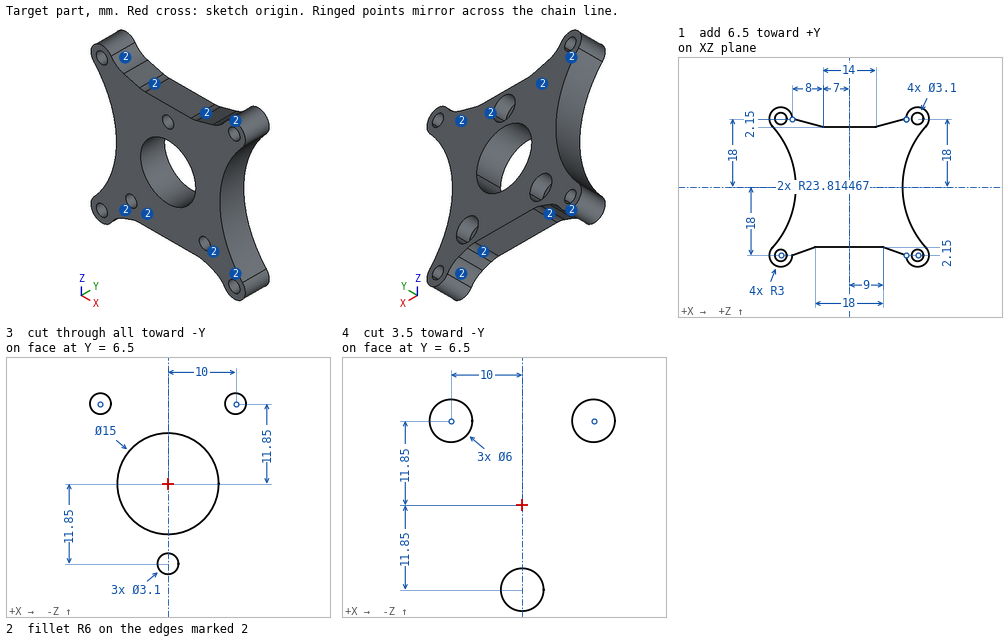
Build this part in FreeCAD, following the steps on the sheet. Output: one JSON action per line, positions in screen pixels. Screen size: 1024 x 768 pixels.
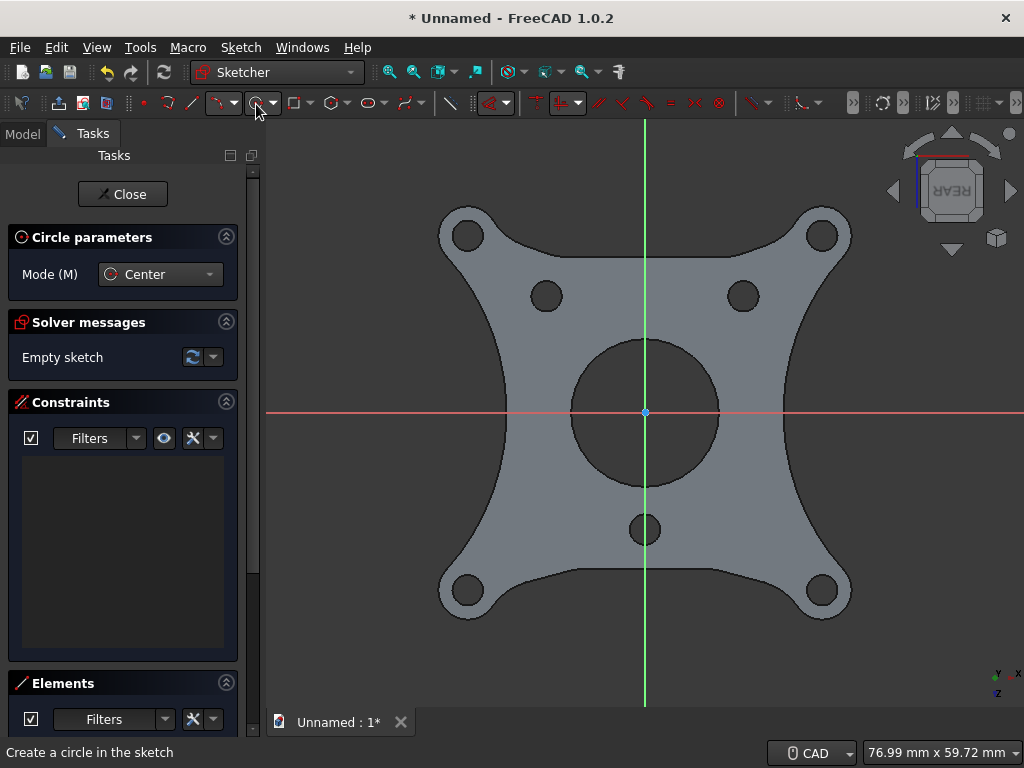
{"action": "left_click", "coordinate": [547, 296]}
{"action": "left_click", "coordinate": [567, 275]}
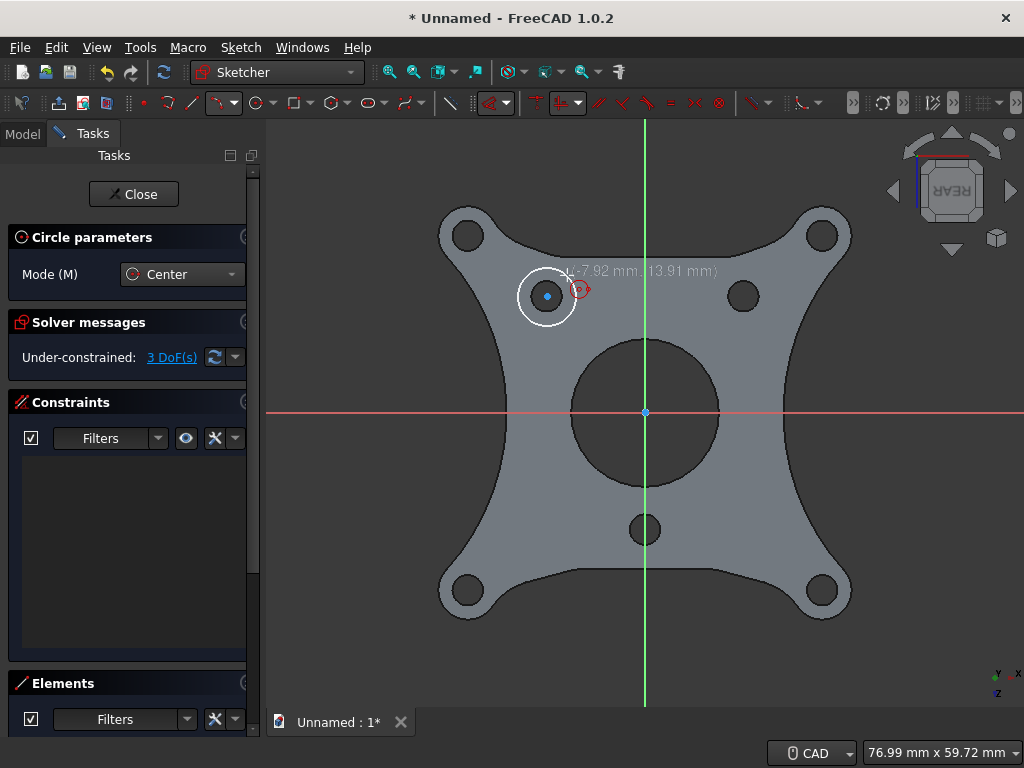
{"action": "left_click", "coordinate": [743, 296]}
{"action": "left_click", "coordinate": [764, 275]}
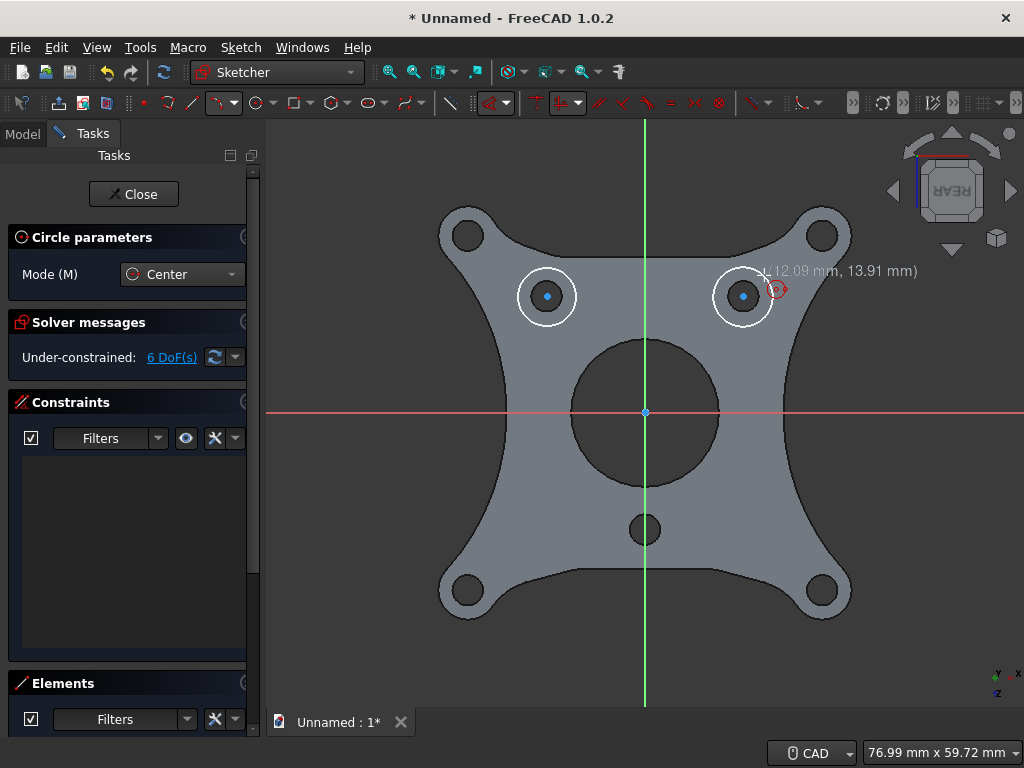
{"action": "left_click", "coordinate": [645, 530]}
{"action": "left_click", "coordinate": [666, 509]}
{"action": "key", "text": "Escape"}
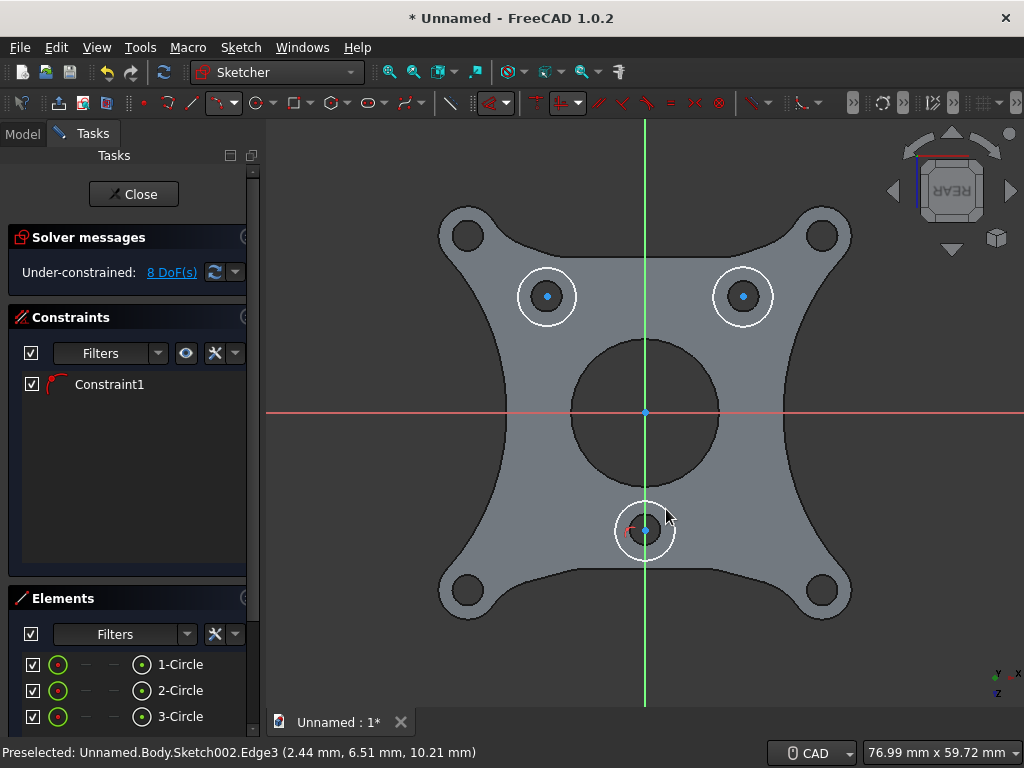
{"action": "left_click", "coordinate": [567, 276]}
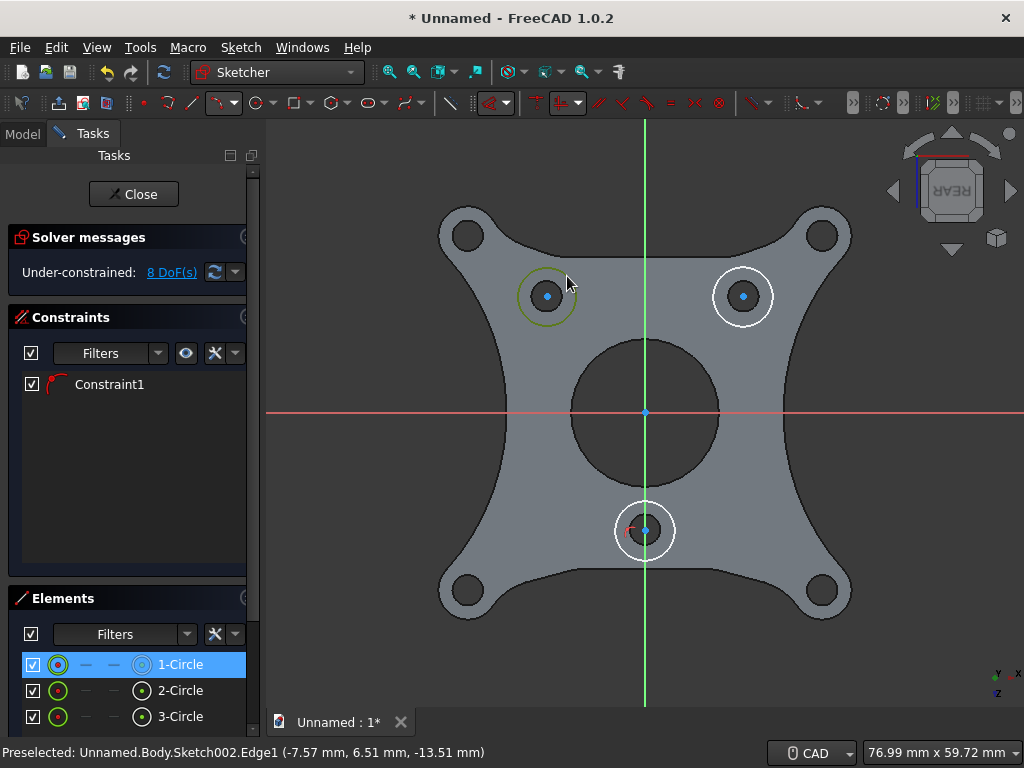
{"action": "left_click", "coordinate": [764, 276]}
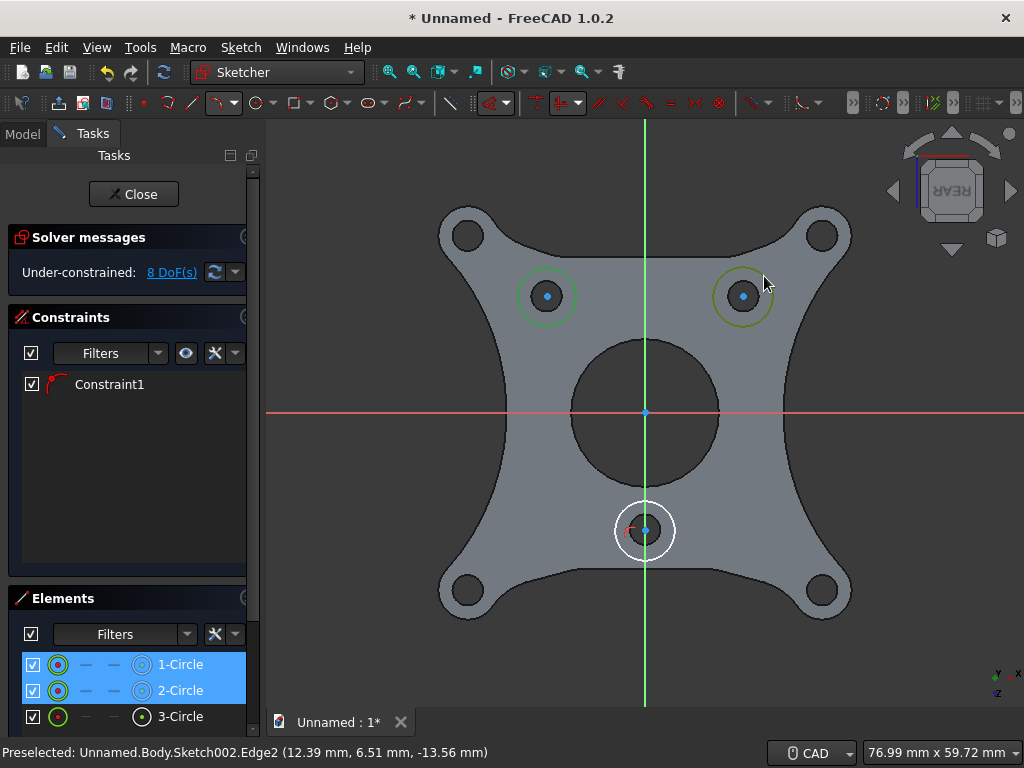
{"action": "left_click", "coordinate": [666, 510]}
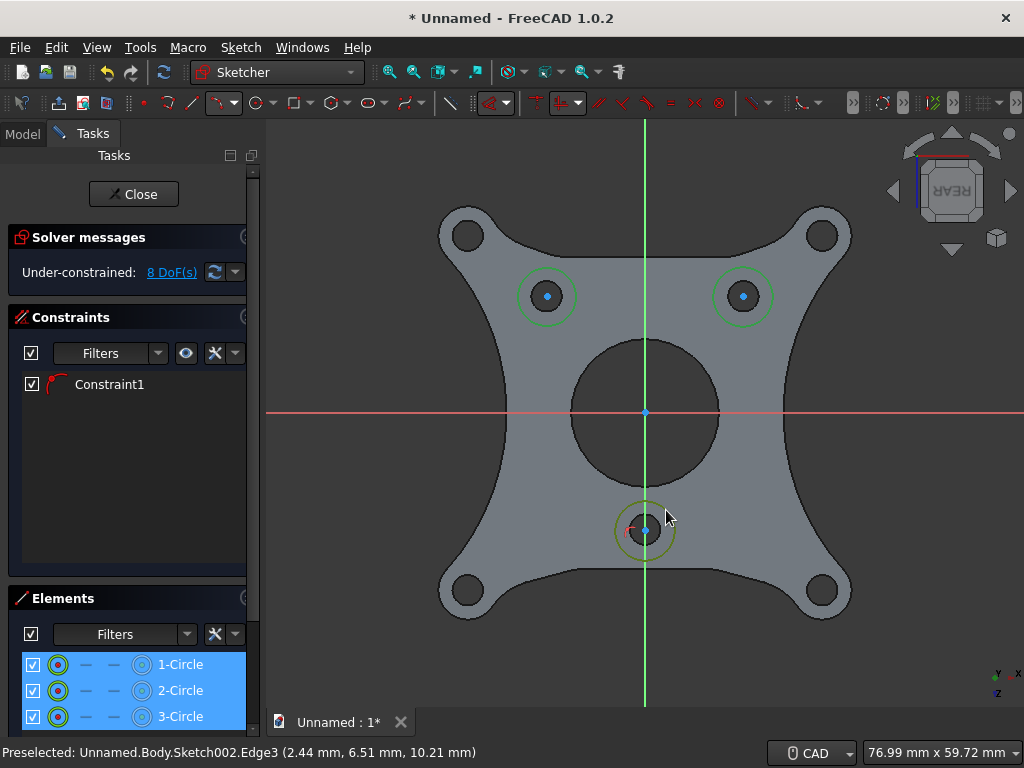
{"action": "left_click", "coordinate": [672, 104]}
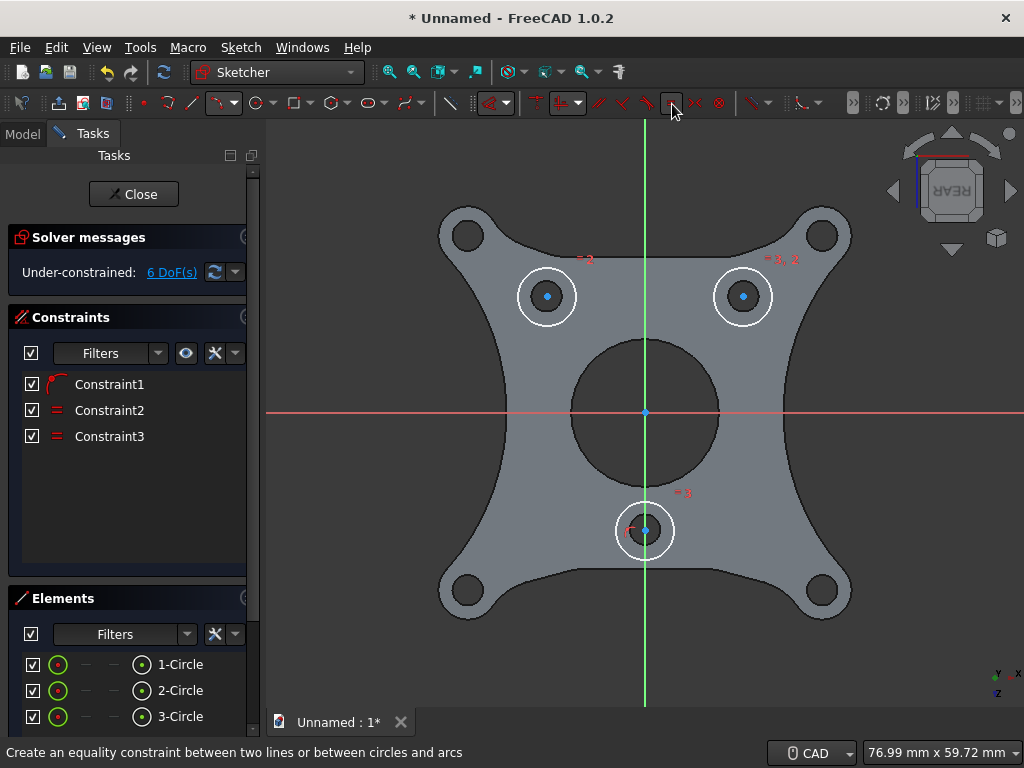
{"action": "left_click", "coordinate": [547, 297]}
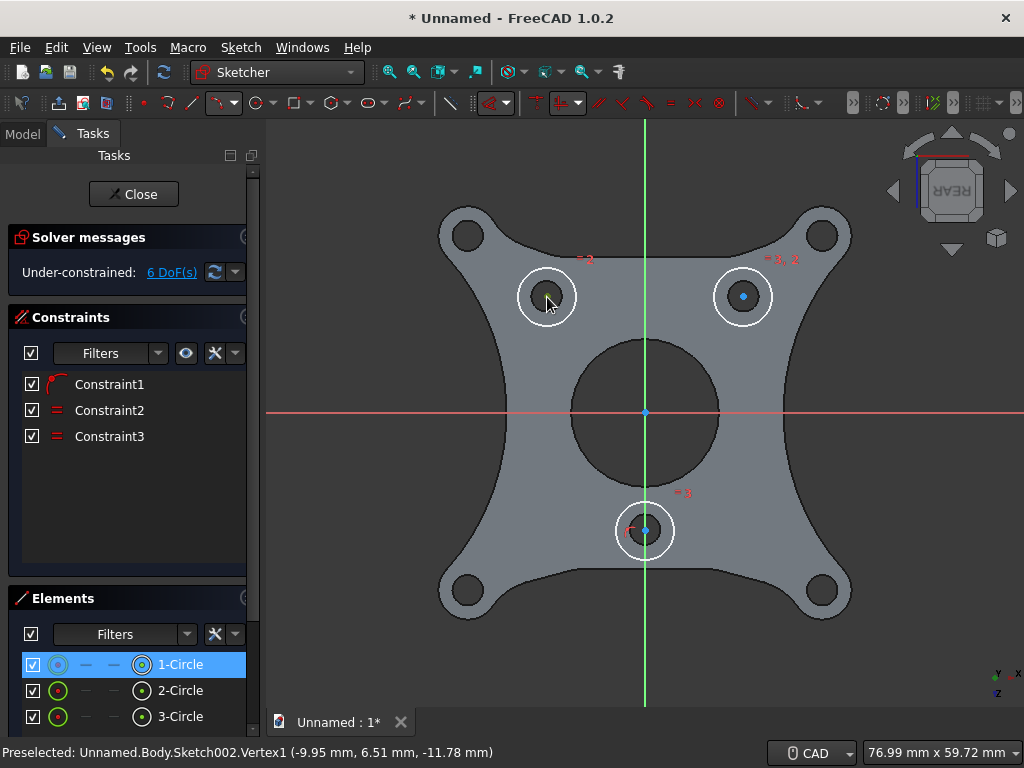
{"action": "left_click", "coordinate": [743, 297]}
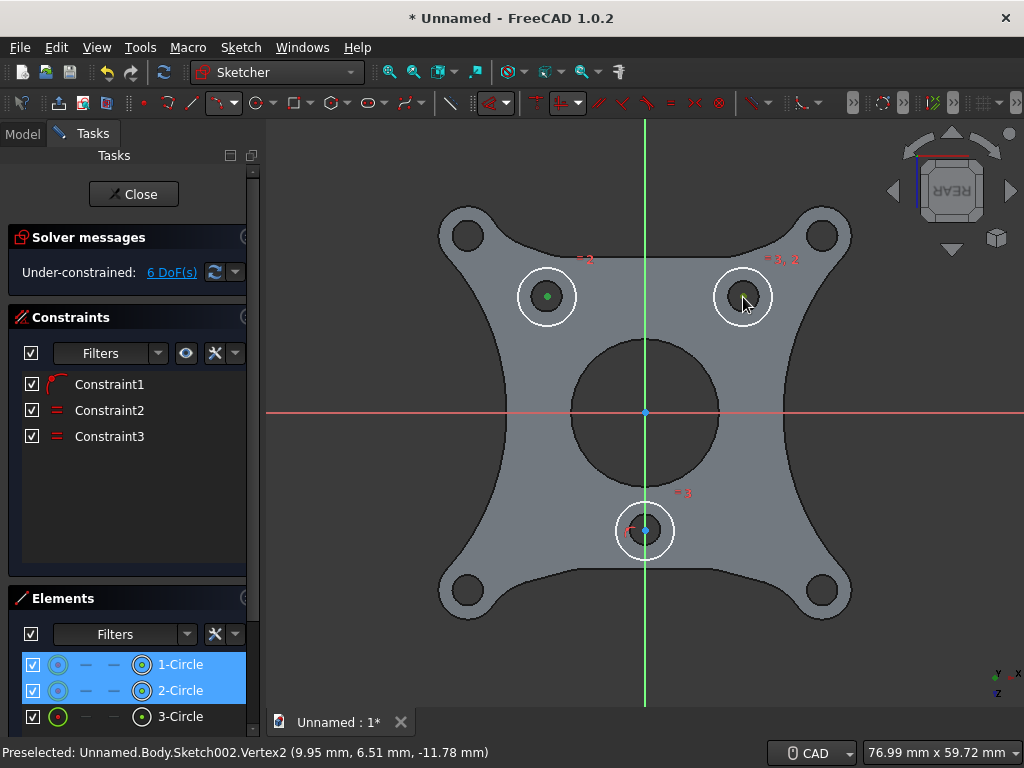
{"action": "left_click", "coordinate": [645, 641]}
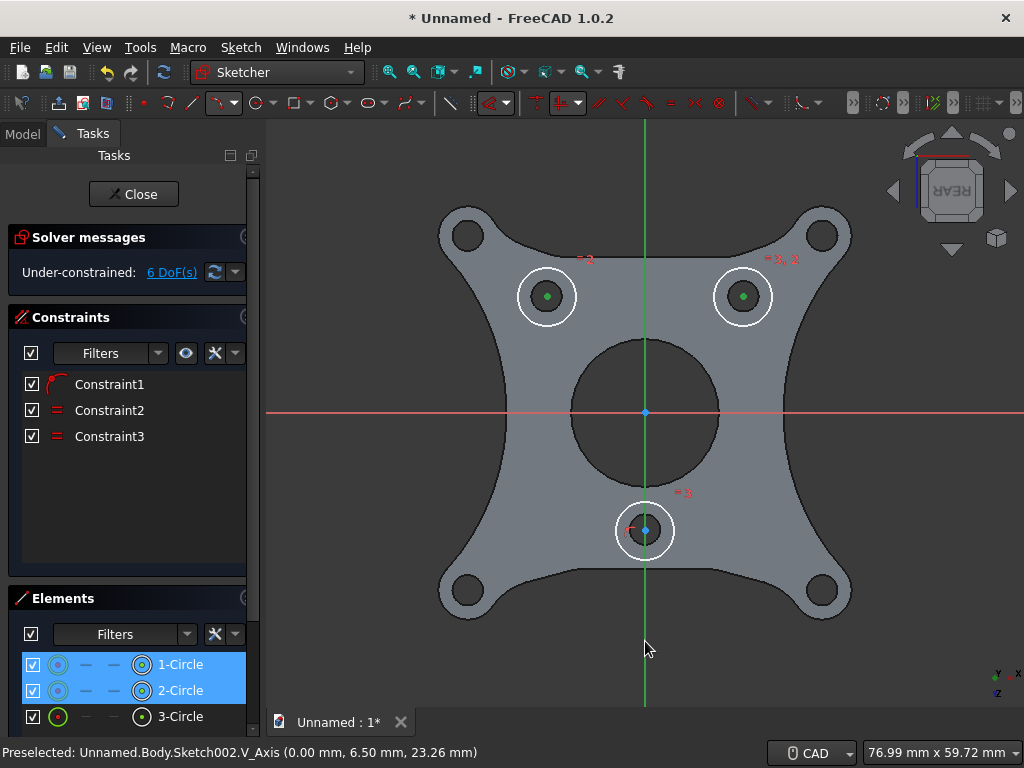
{"action": "left_click", "coordinate": [696, 104]}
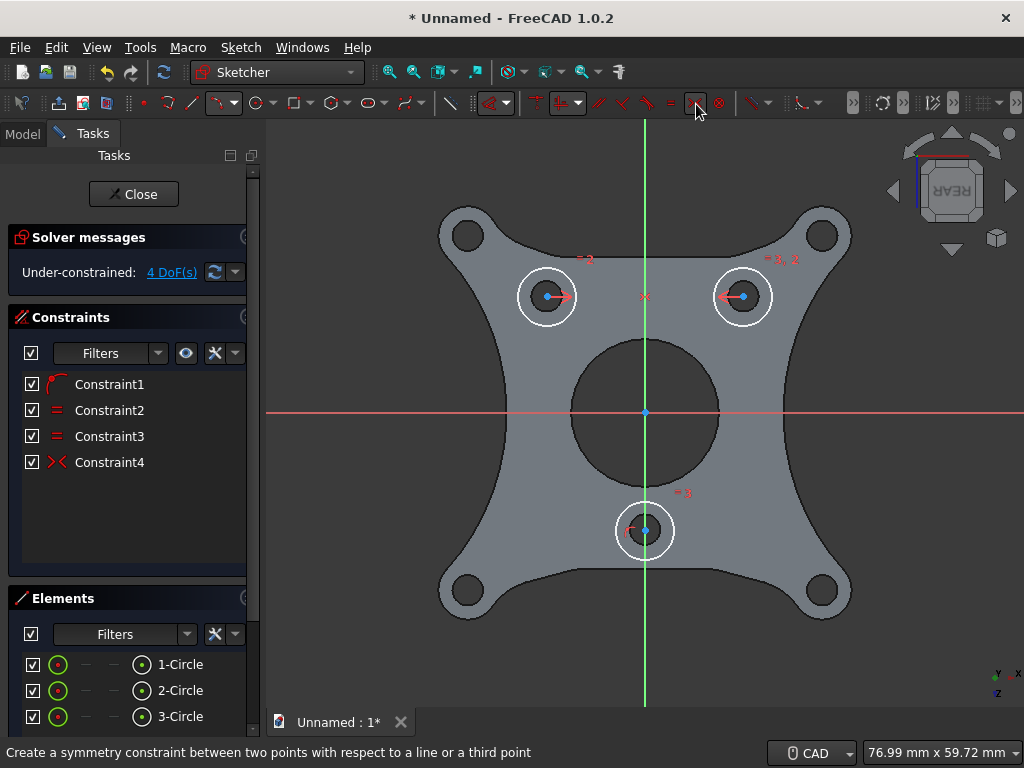
{"action": "left_click", "coordinate": [567, 276]}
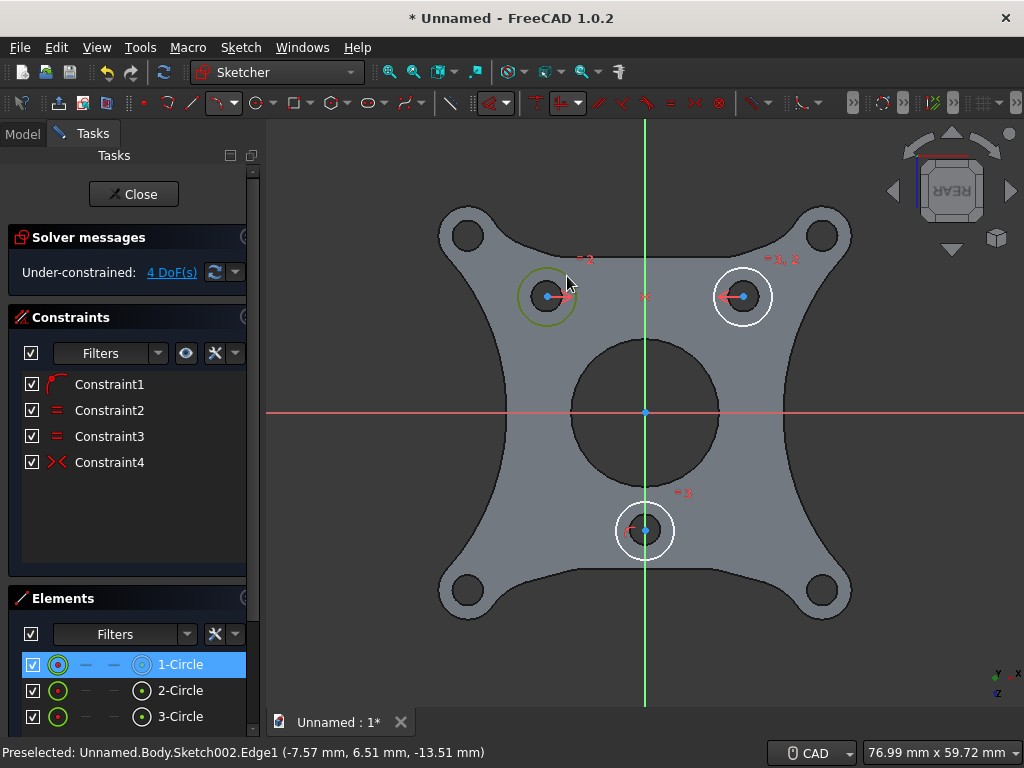
{"action": "key", "text": "k o"}